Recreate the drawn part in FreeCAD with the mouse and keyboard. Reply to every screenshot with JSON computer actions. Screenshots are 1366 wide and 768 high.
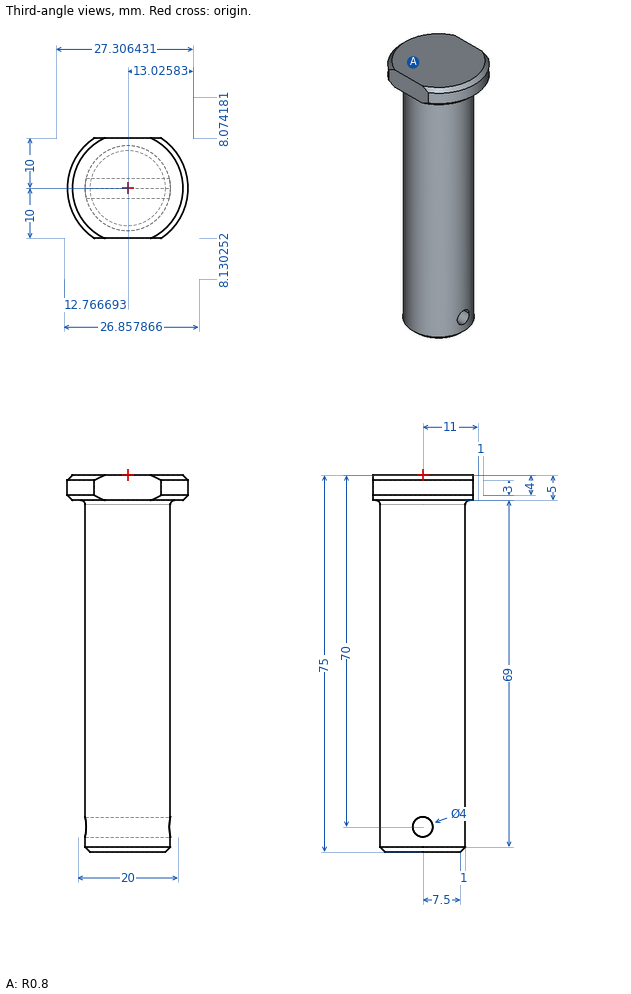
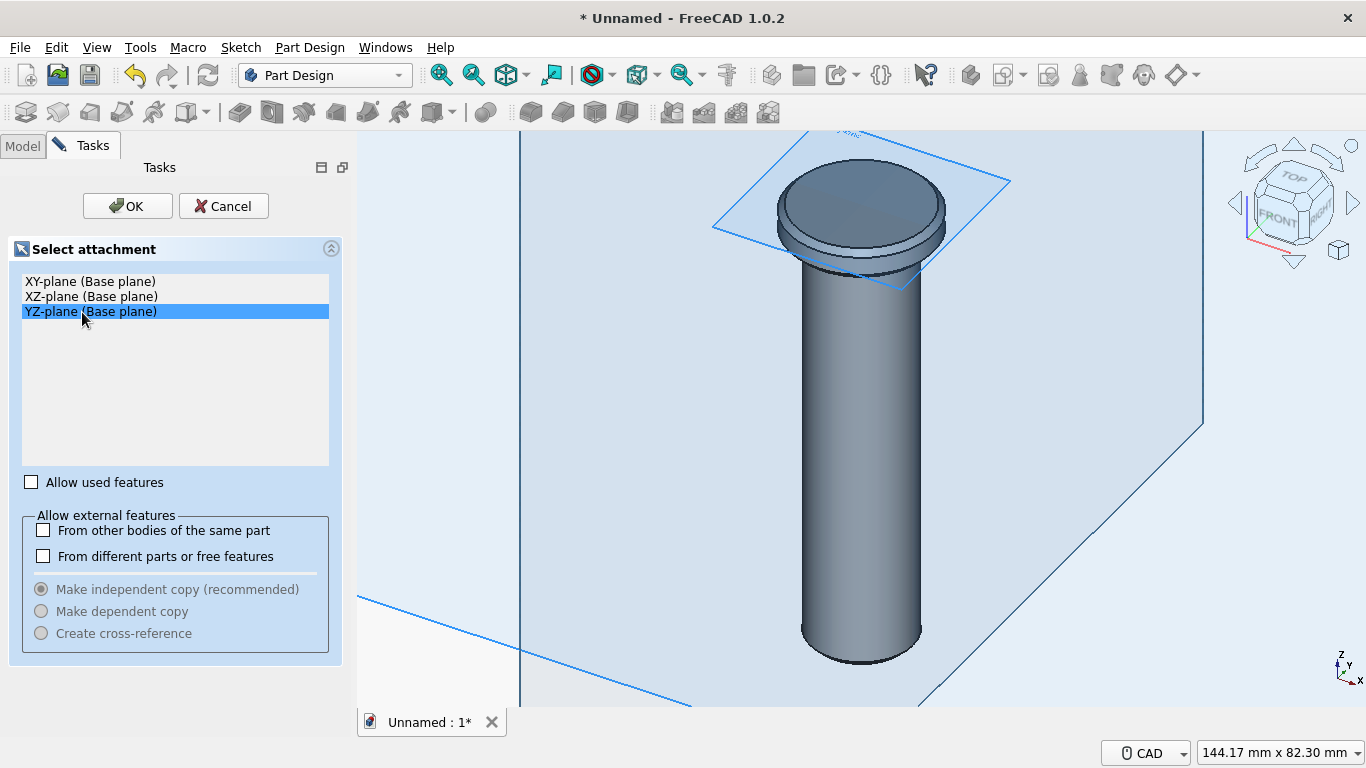
{"action": "left_click", "coordinate": [128, 206]}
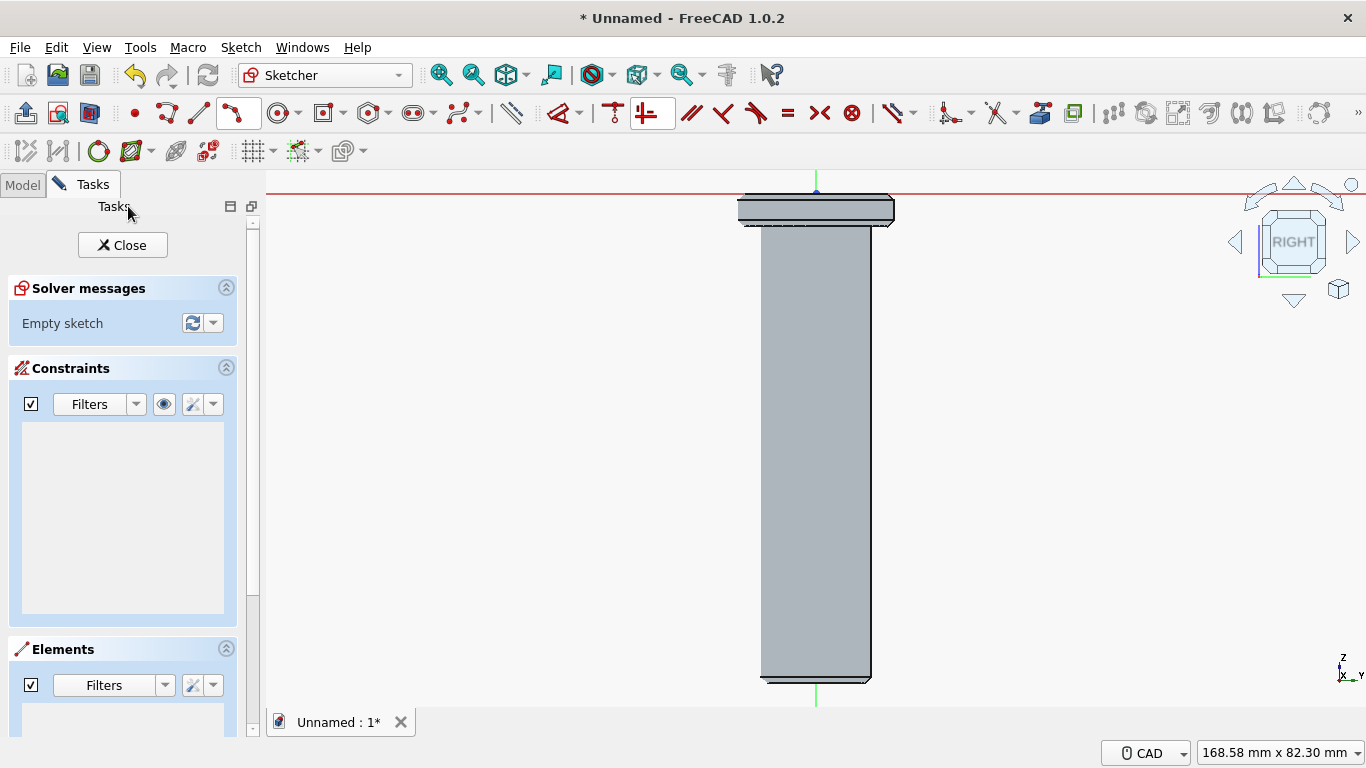
{"action": "left_click", "coordinate": [90, 114]}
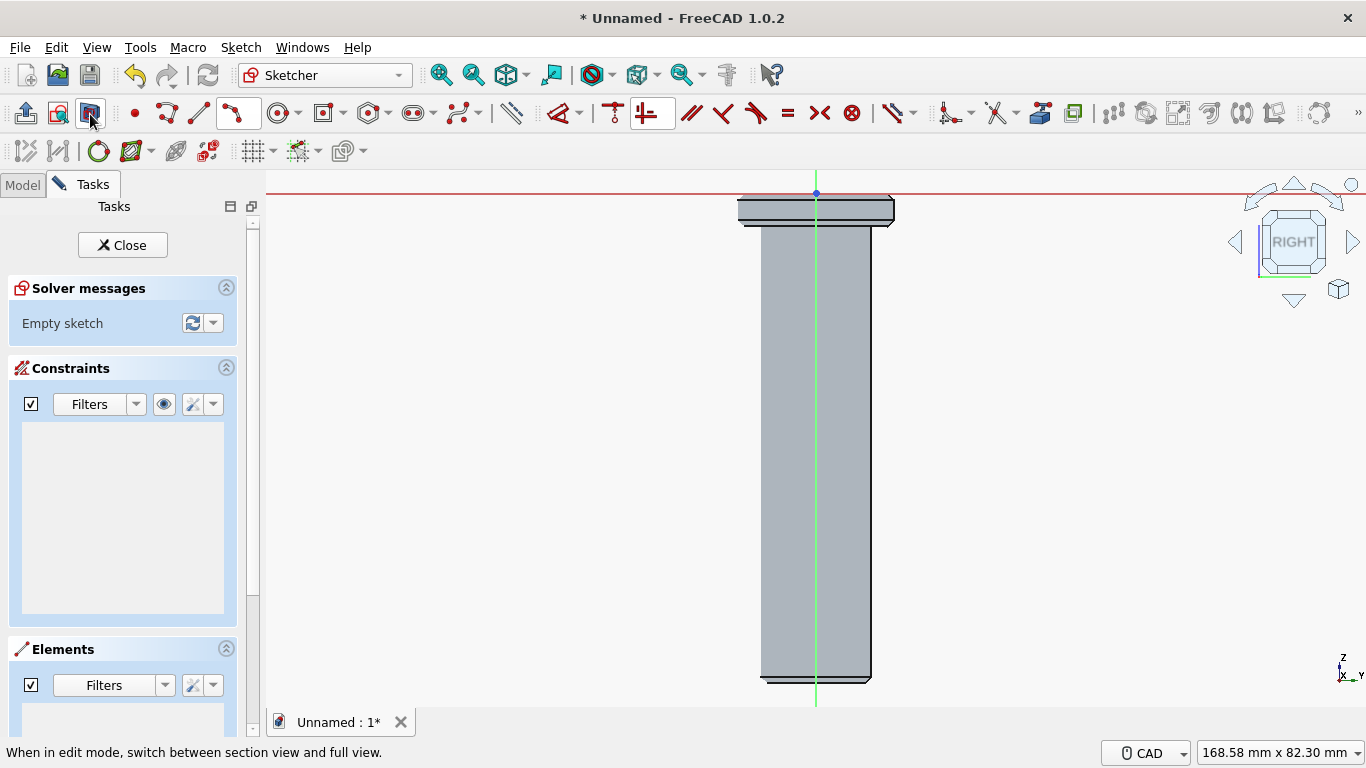
{"action": "scroll", "coordinate": [821, 668], "scroll_direction": "up", "scroll_amount": 13}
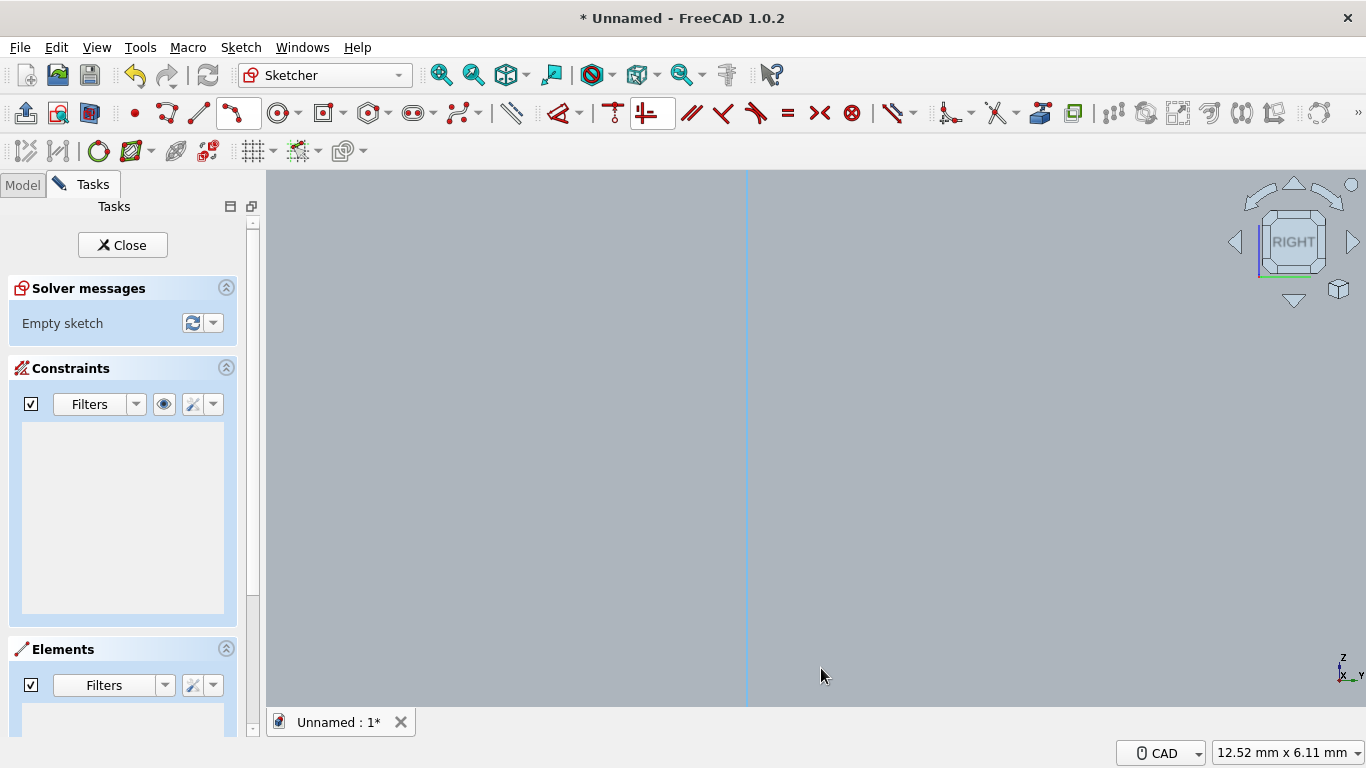
{"action": "key", "text": "g c"}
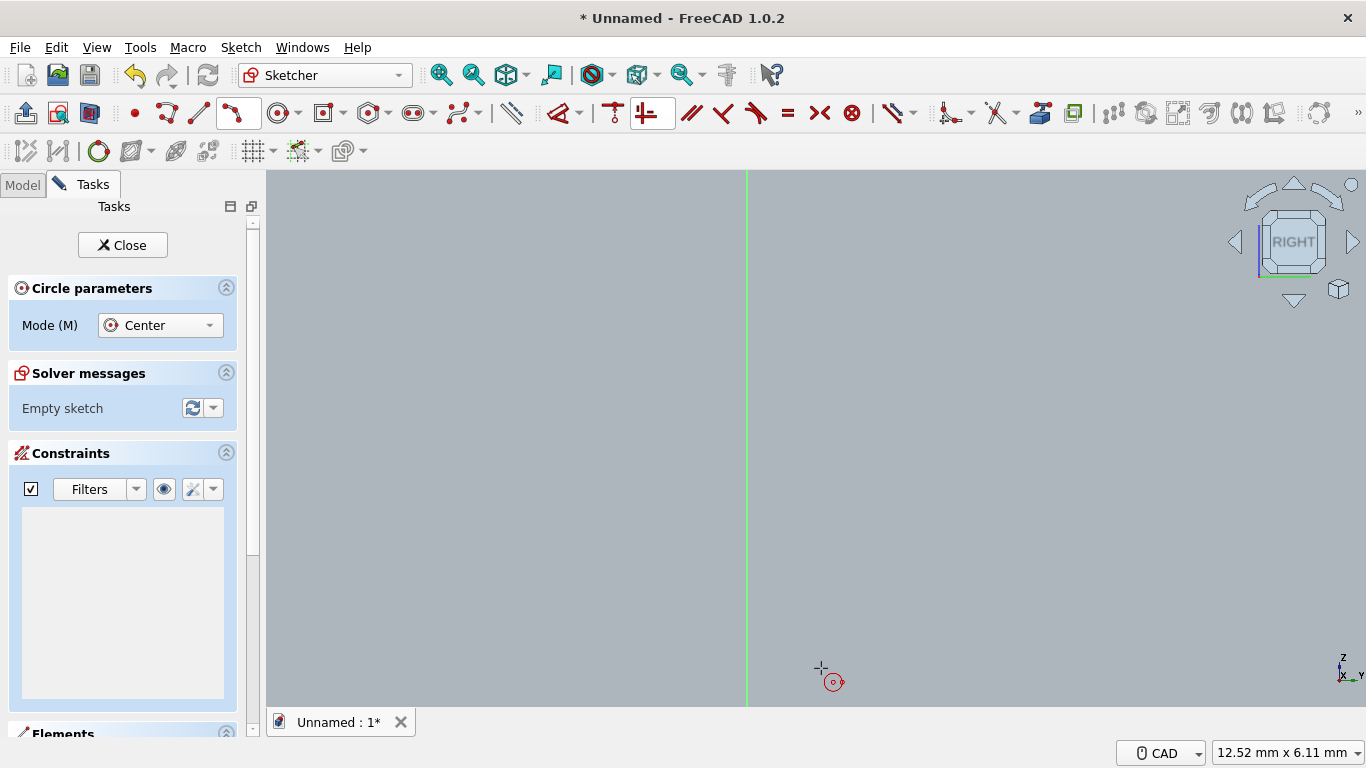
{"action": "left_click", "coordinate": [747, 422]}
{"action": "mouse_move", "coordinate": [872, 297]}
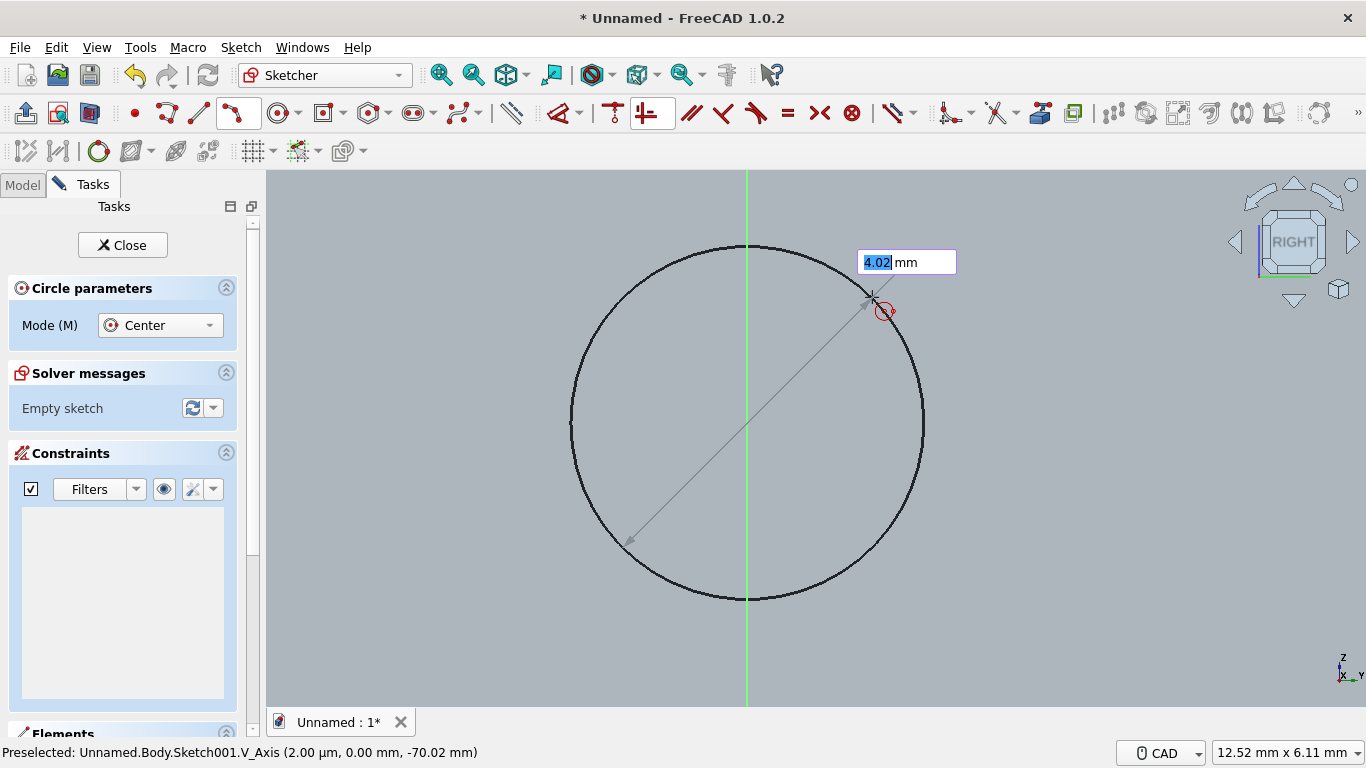
{"action": "type", "text": "4"}
{"action": "key", "text": "Return"}
{"action": "key", "text": "Escape"}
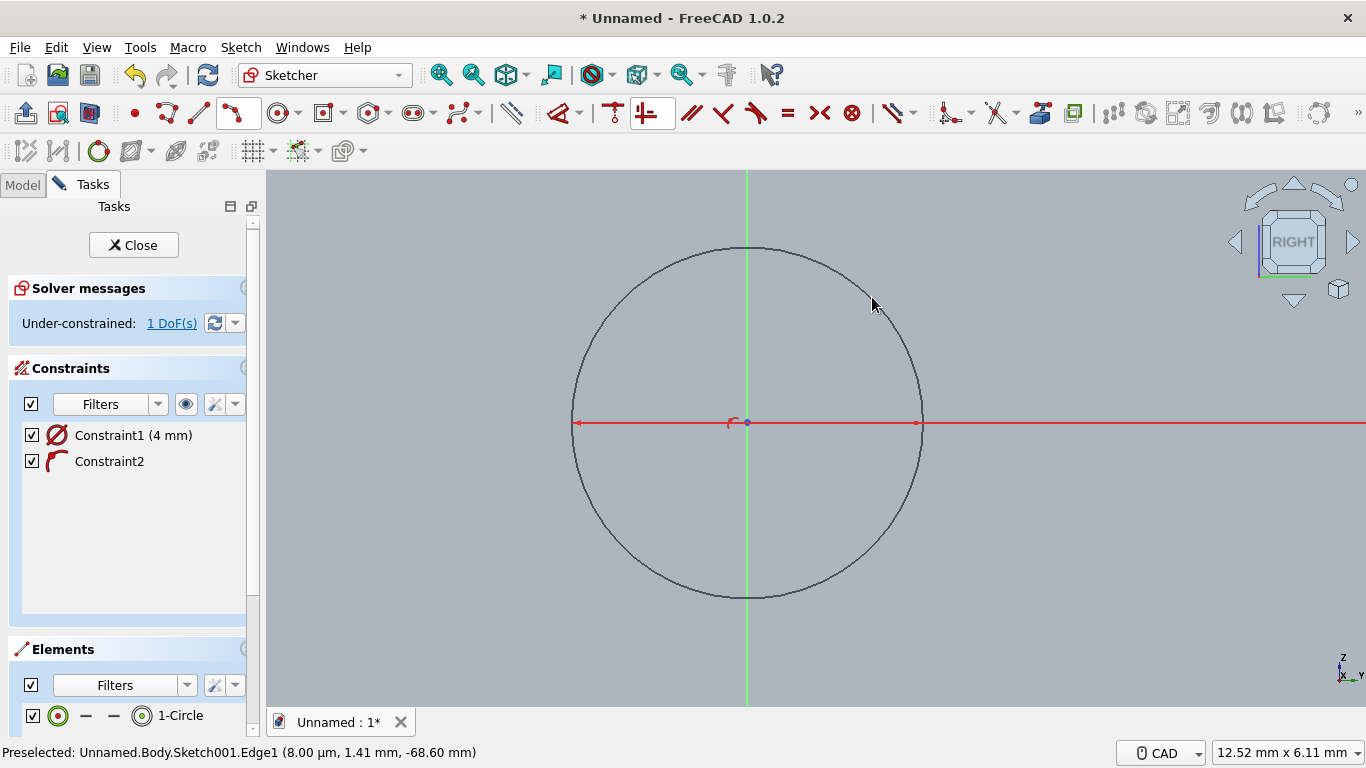
{"action": "left_click", "coordinate": [558, 114]}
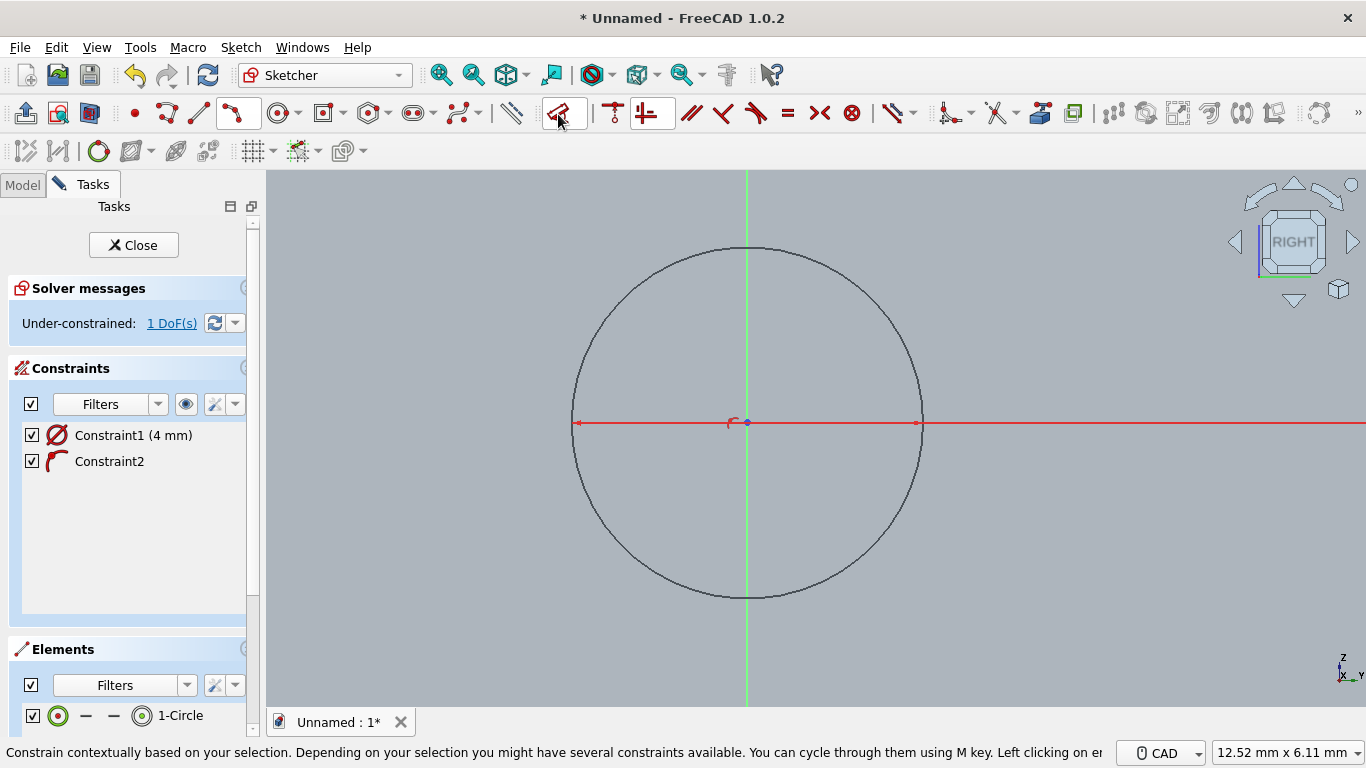
{"action": "left_click", "coordinate": [747, 423]}
{"action": "left_click", "coordinate": [781, 310]}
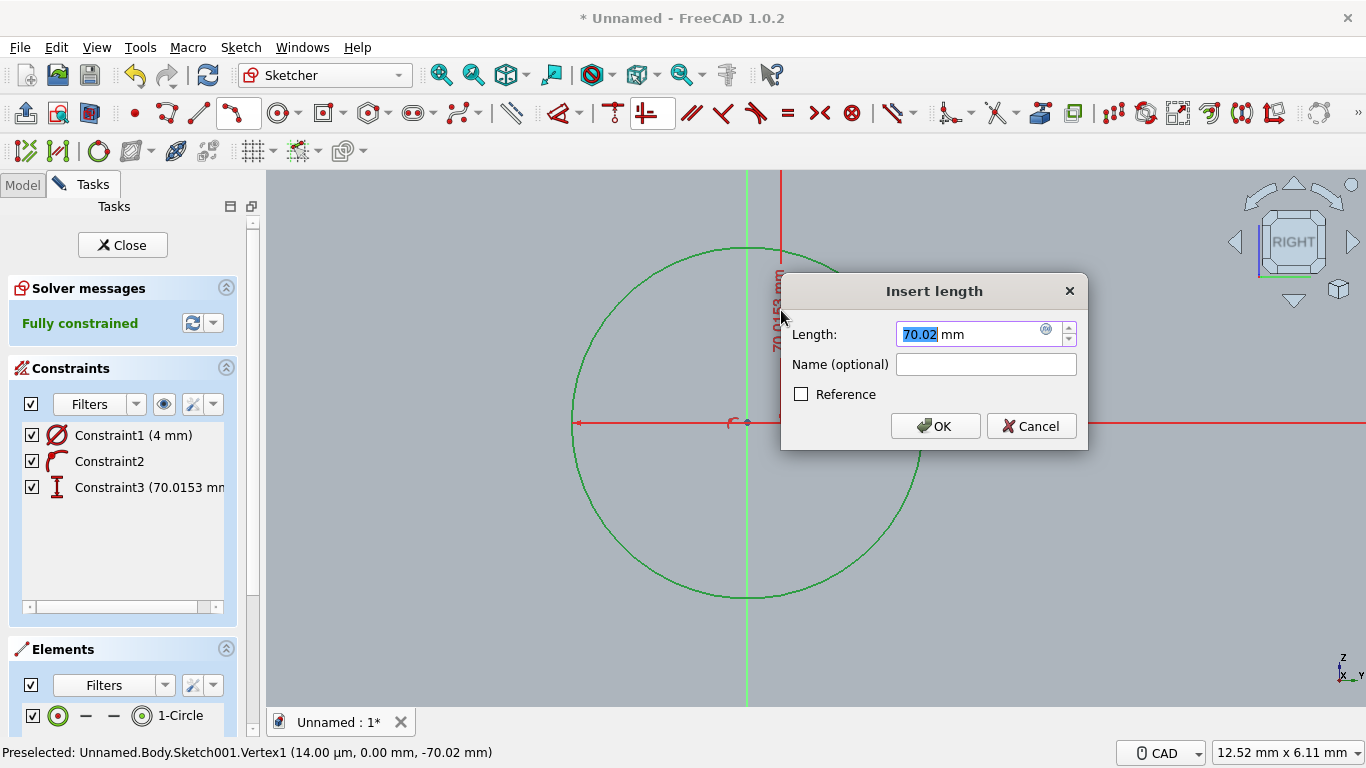
{"action": "type", "text": "70"}
{"action": "key", "text": "Return"}
{"action": "key", "text": "Escape"}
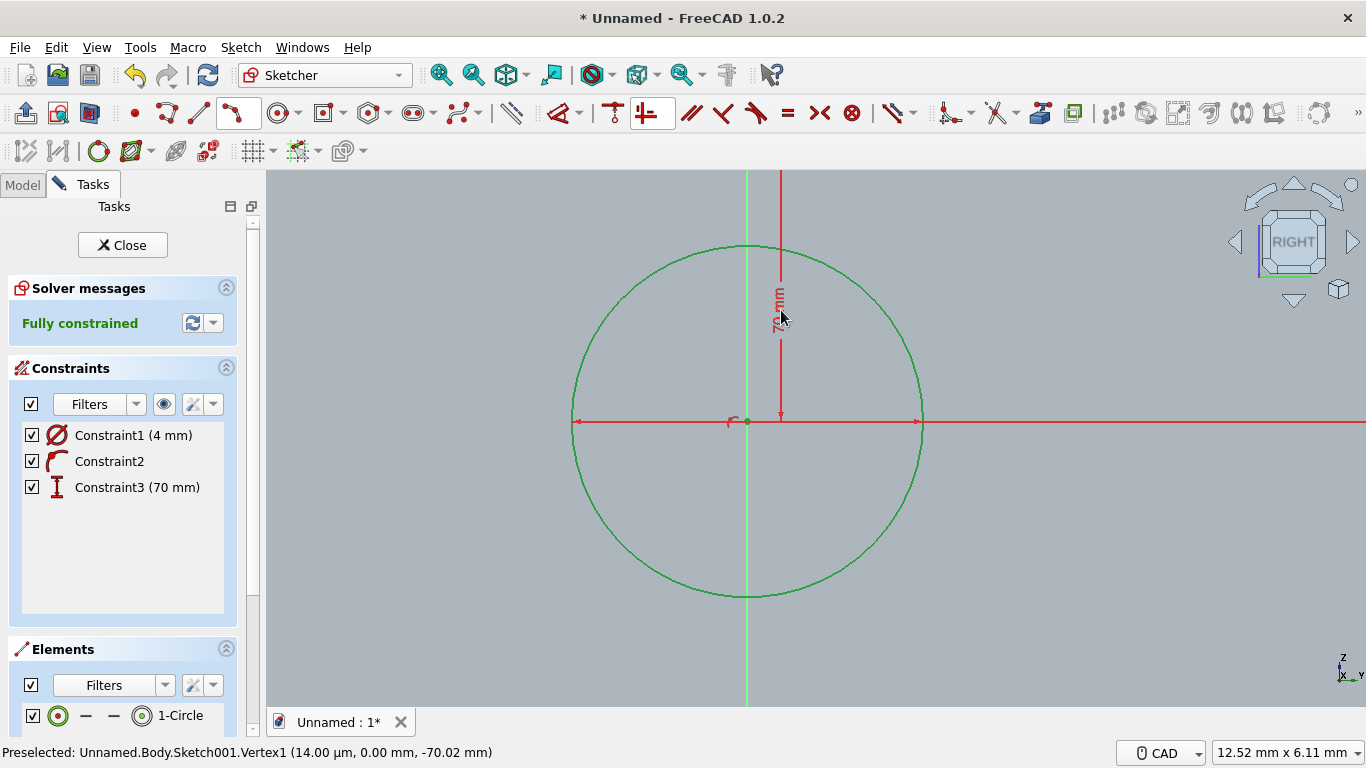
{"action": "left_click", "coordinate": [123, 245]}